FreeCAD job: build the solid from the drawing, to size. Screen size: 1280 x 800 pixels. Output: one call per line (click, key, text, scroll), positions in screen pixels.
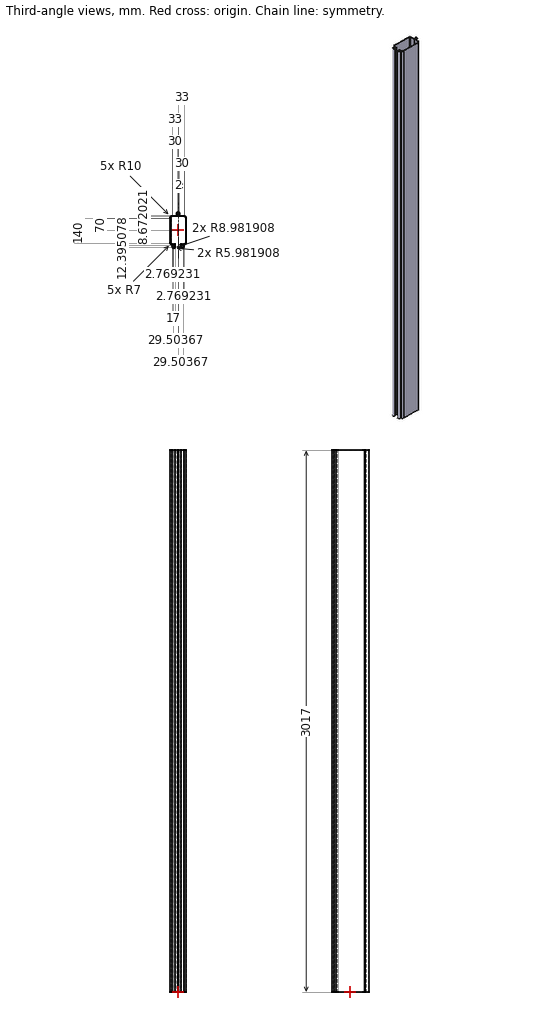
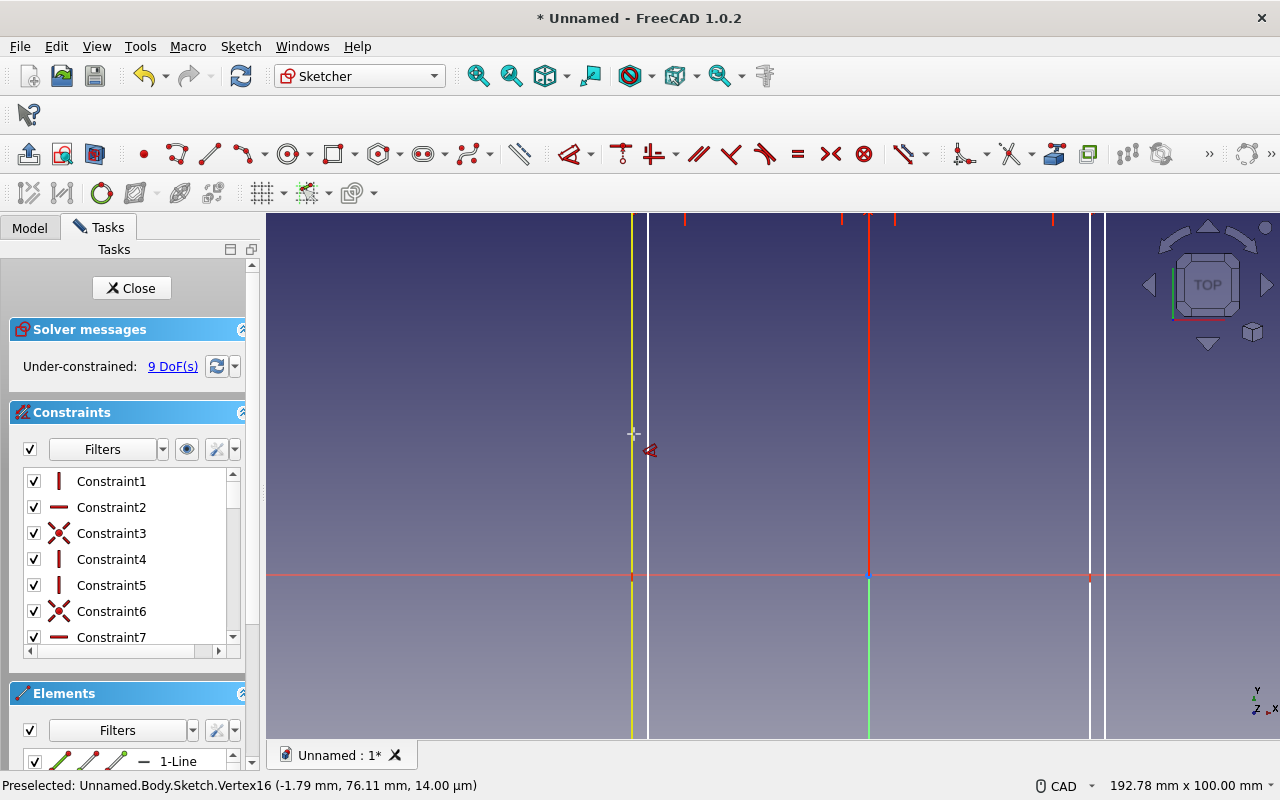
click(632, 432)
click(598, 476)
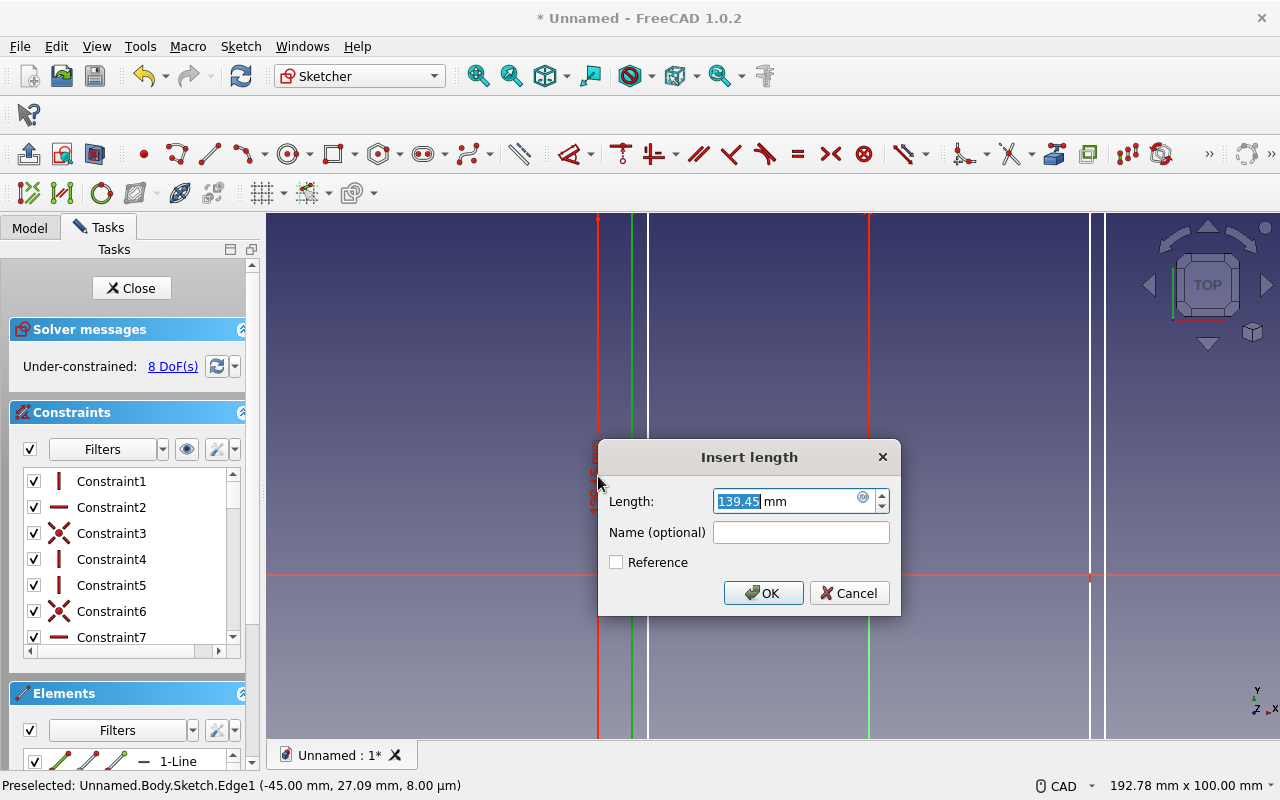
text(140)
key(Return)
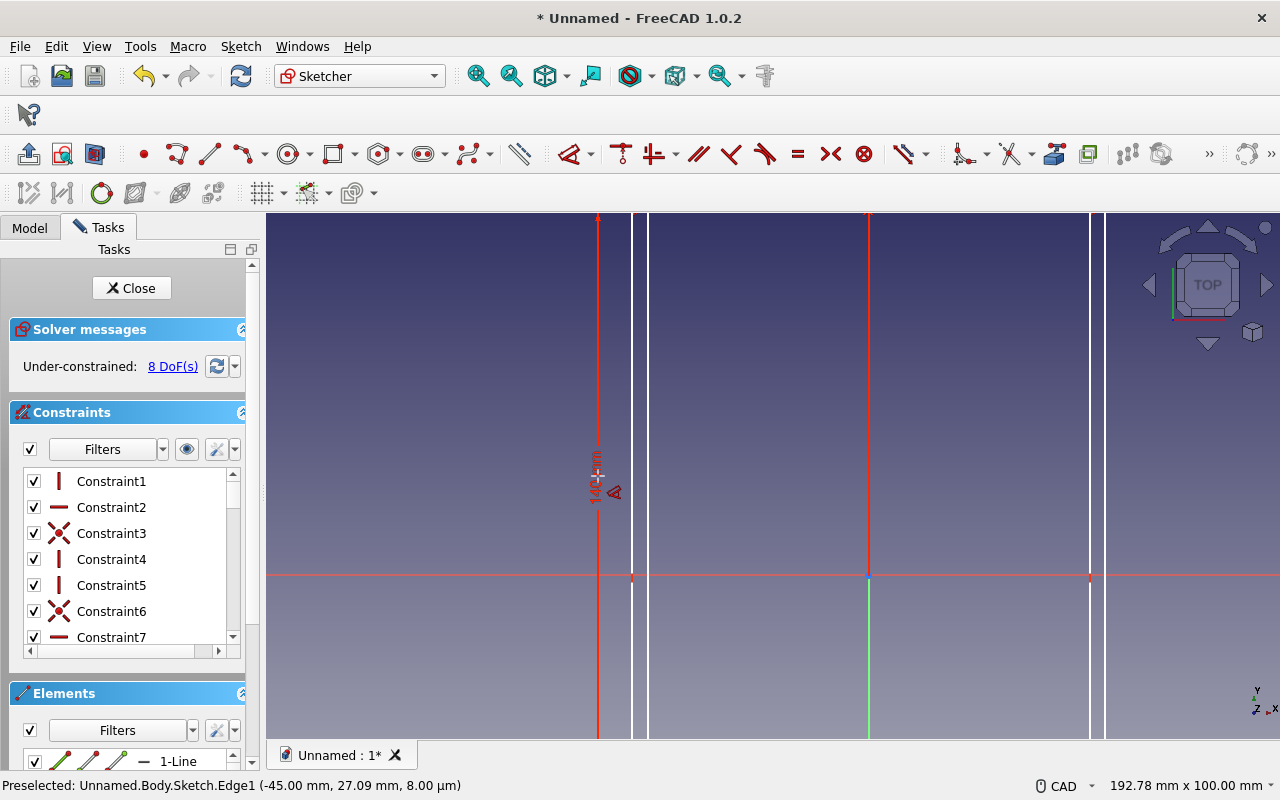
click(1090, 432)
click(1056, 476)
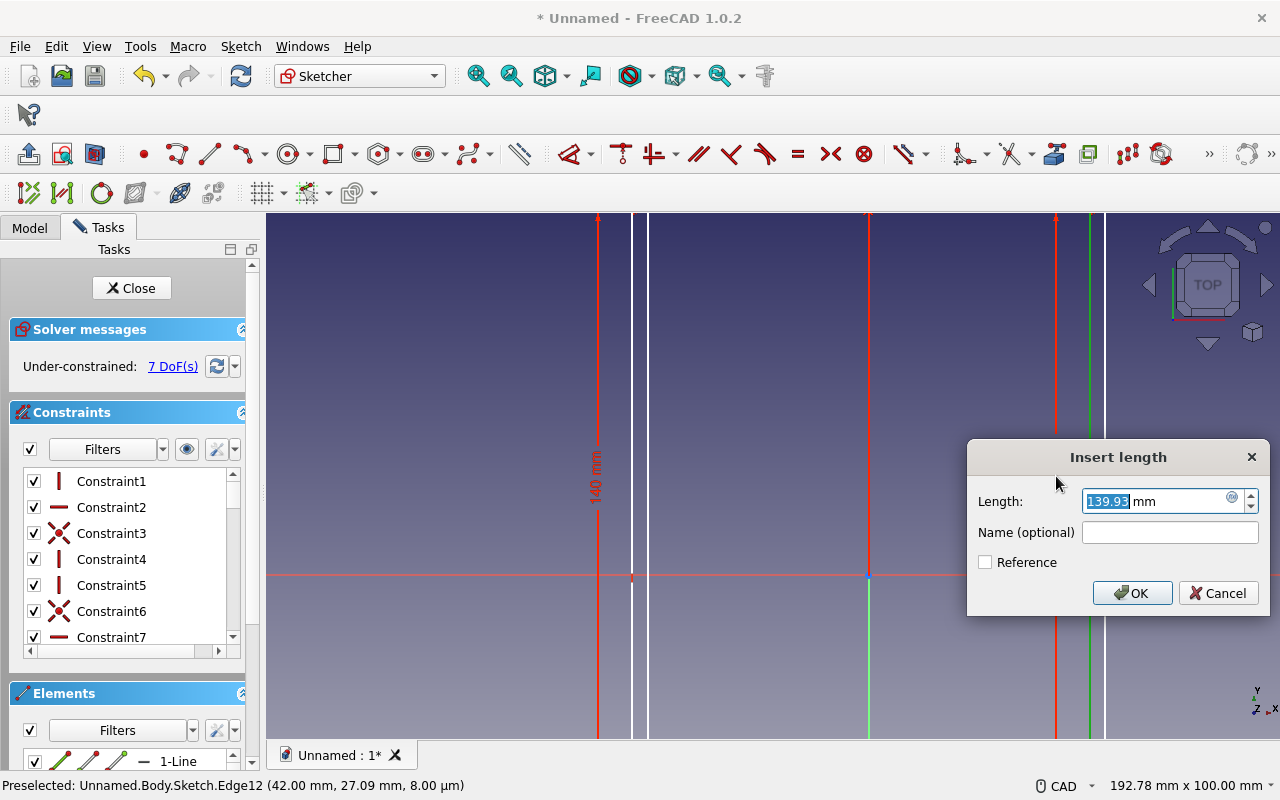
text(140)
key(Return)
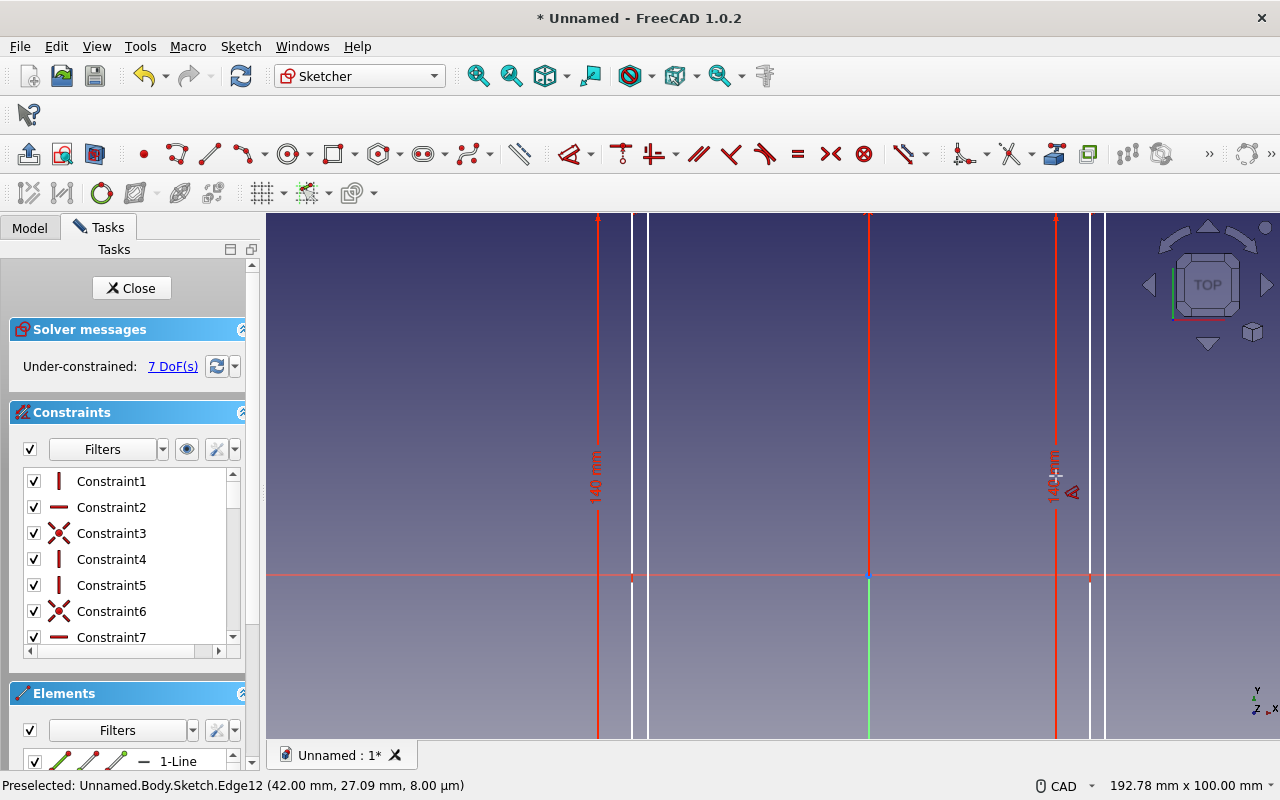
scroll(634, 434, down, 6)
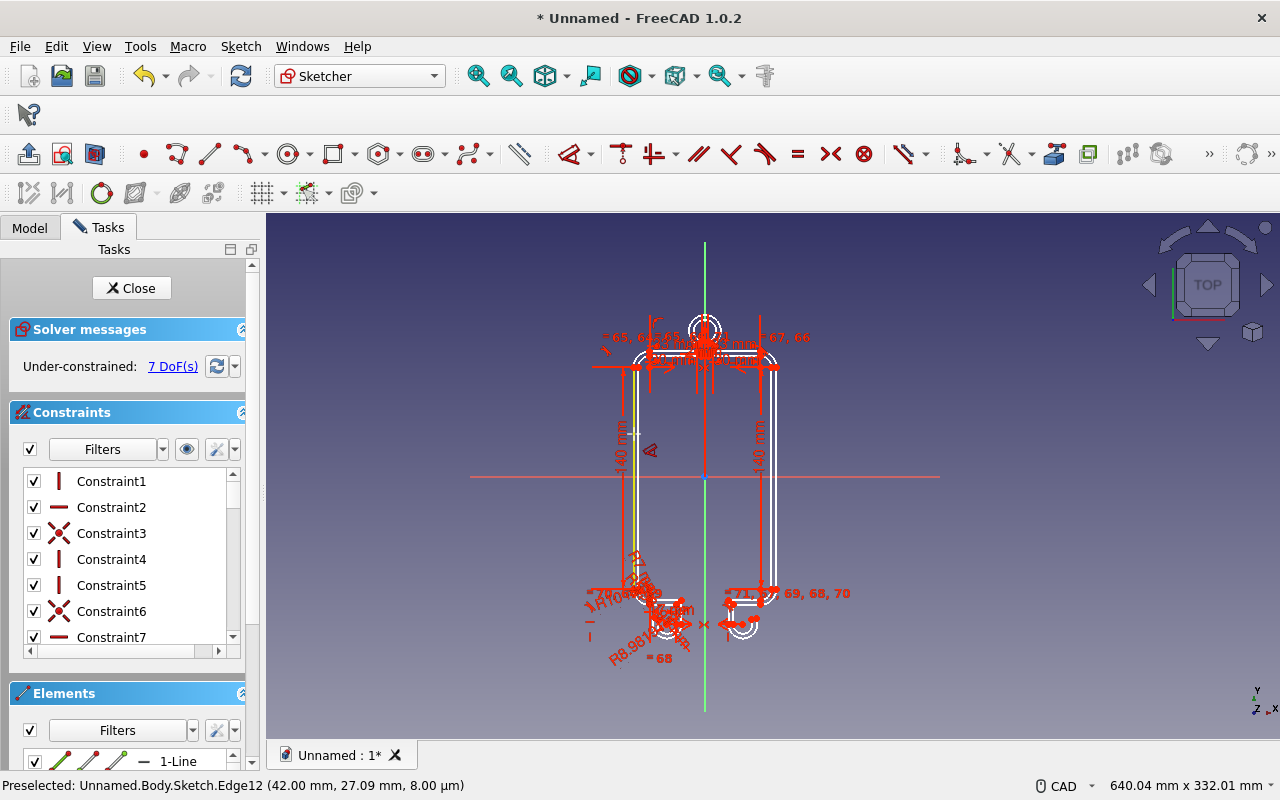
scroll(634, 367, up, 5)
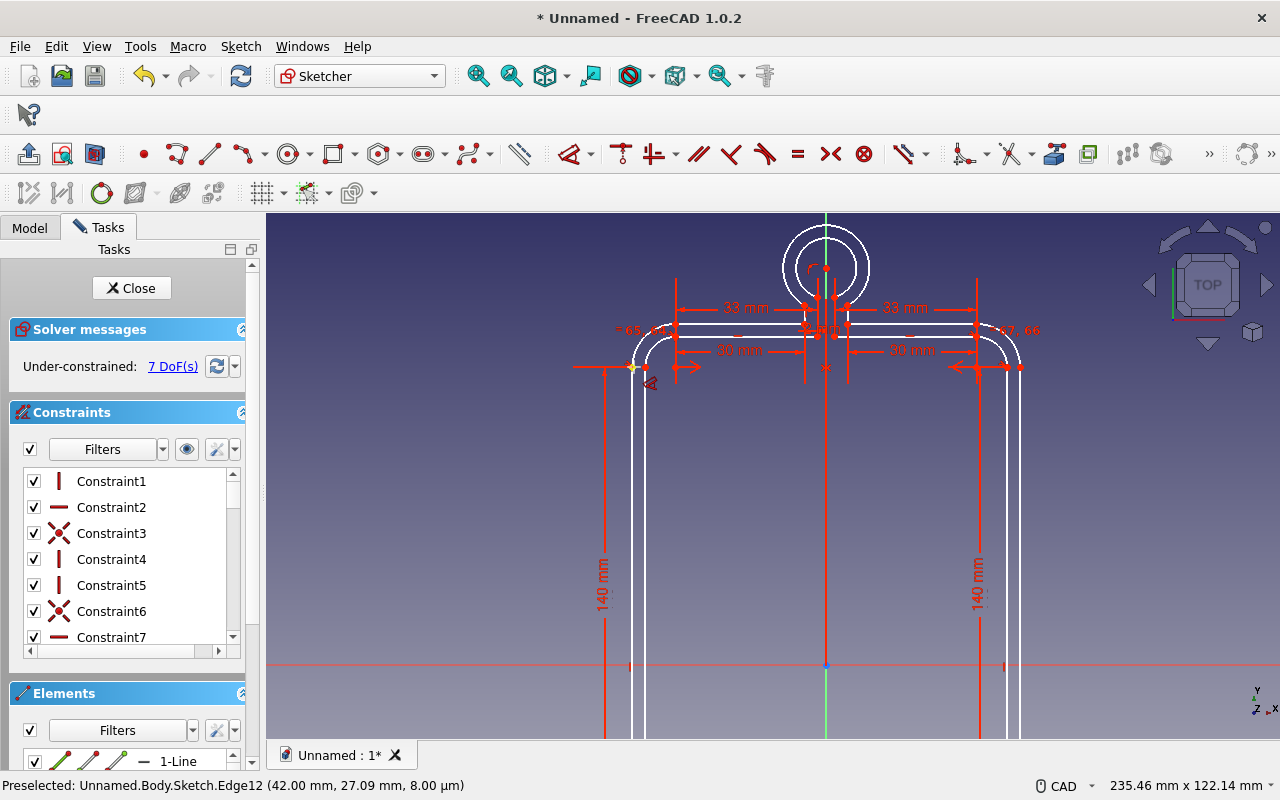
click(632, 367)
click(598, 516)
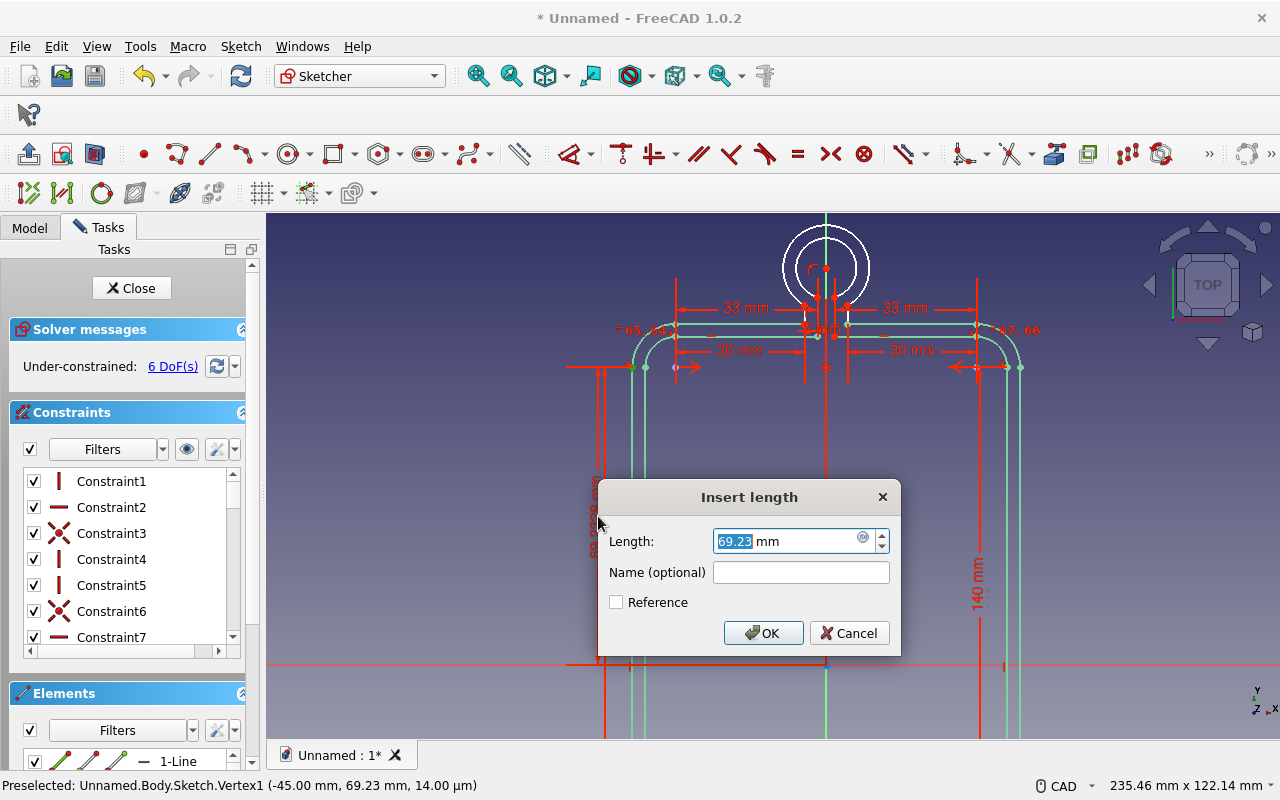
text(70)
key(Return)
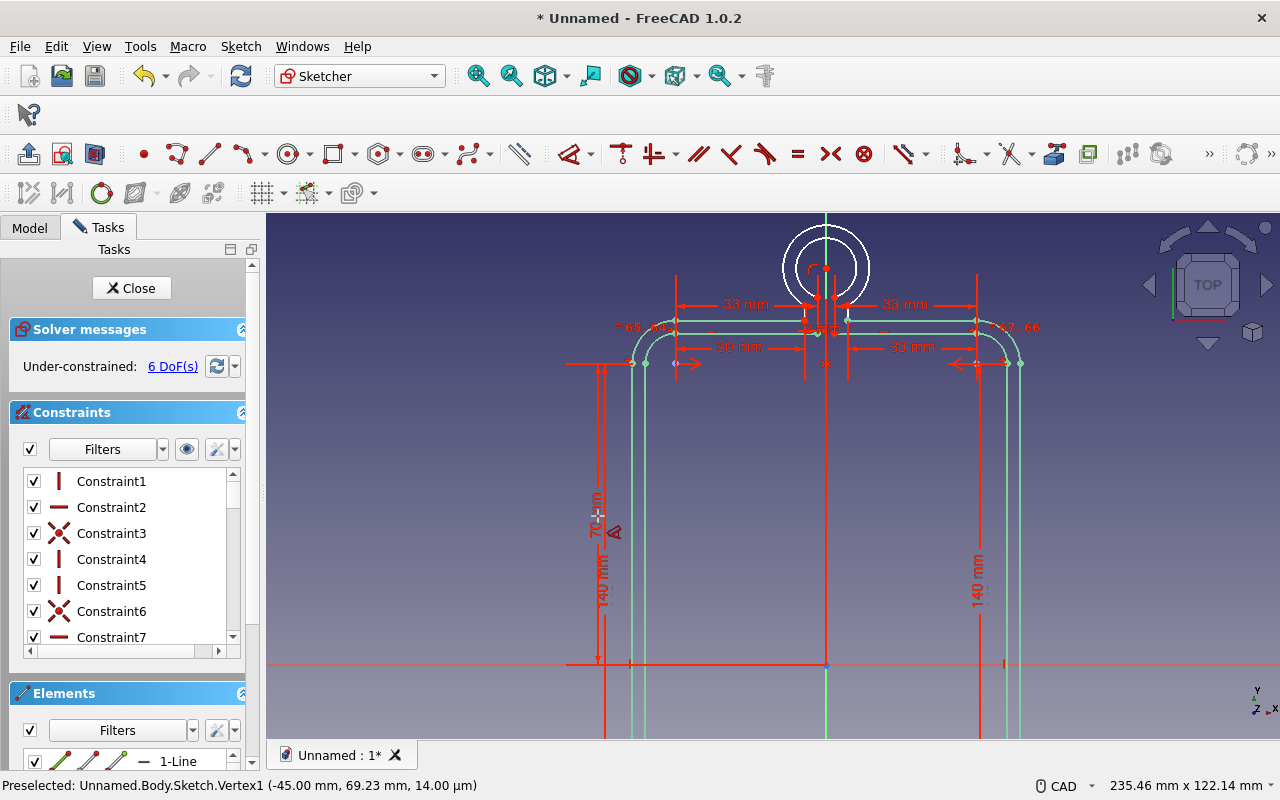
scroll(818, 323, up, 3)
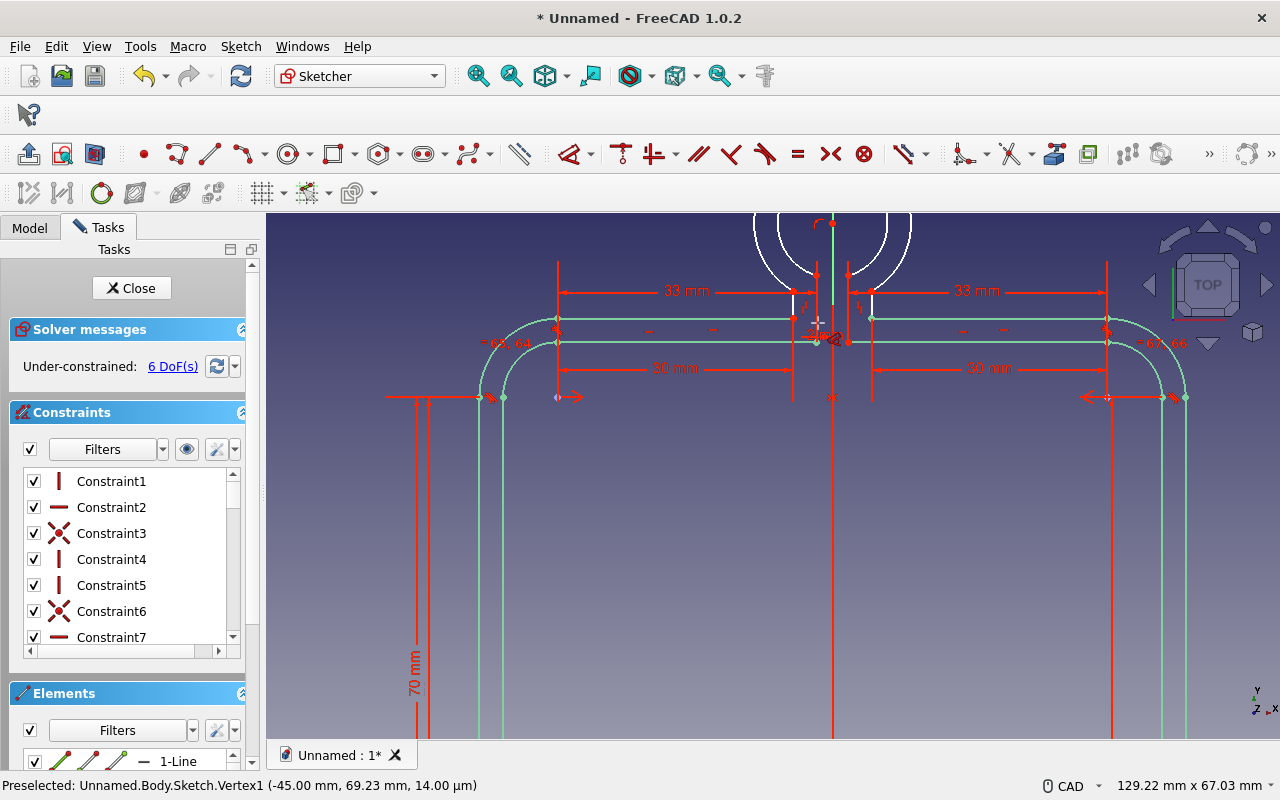
click(817, 322)
click(759, 294)